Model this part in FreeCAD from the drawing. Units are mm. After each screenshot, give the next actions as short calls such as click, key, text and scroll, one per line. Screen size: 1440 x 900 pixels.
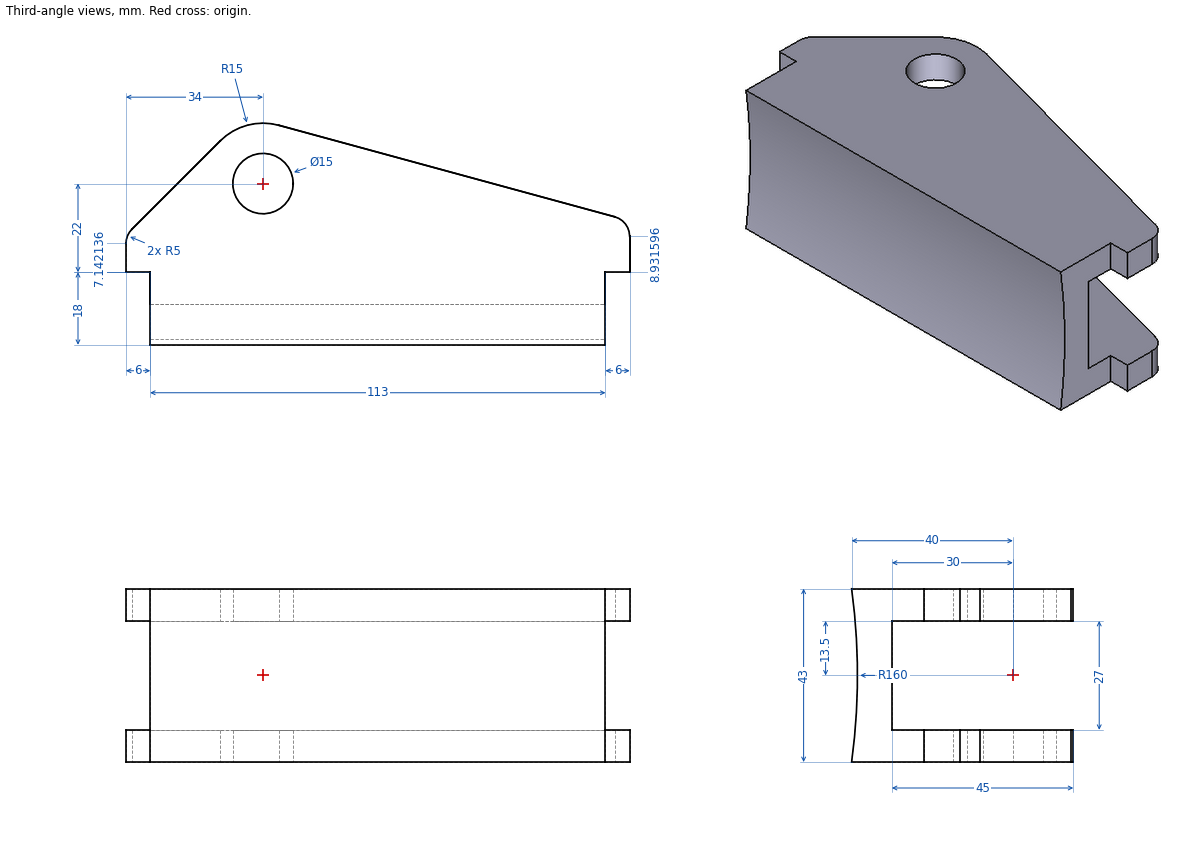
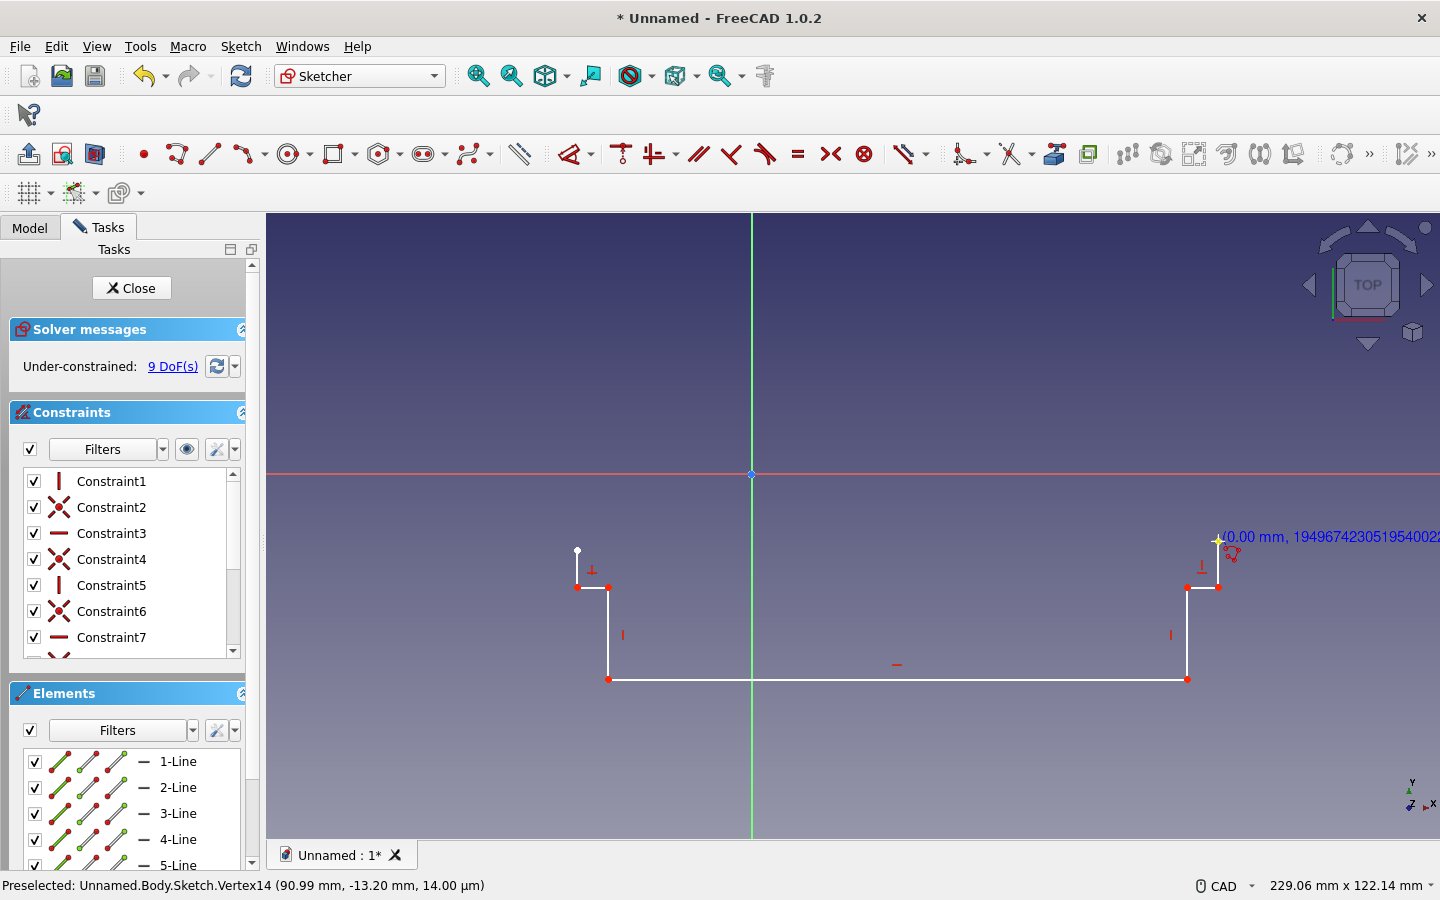
key(g)
key(l)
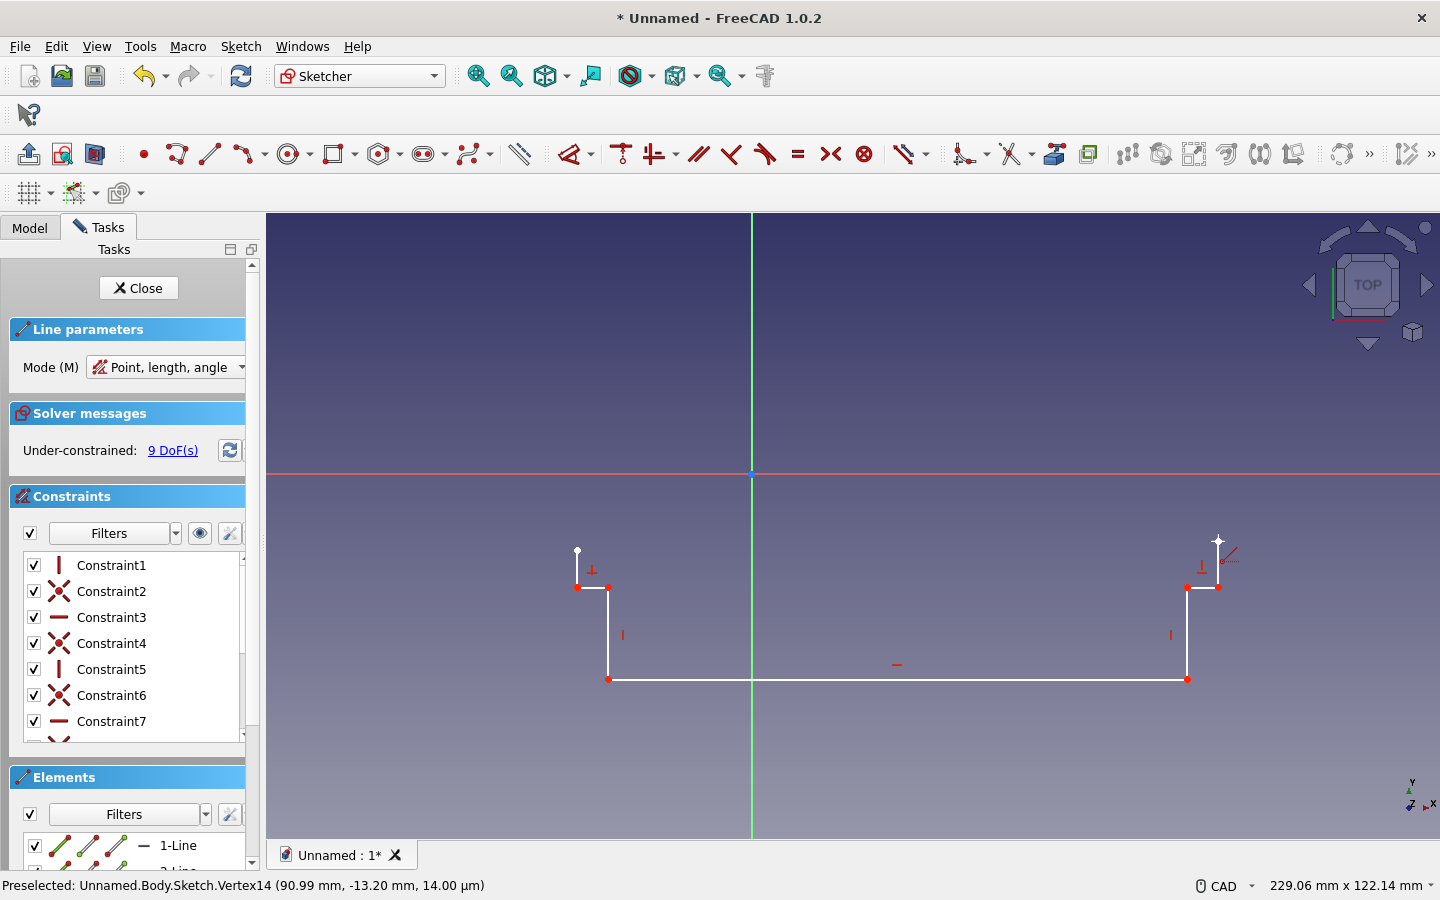
click(1199, 517)
click(772, 400)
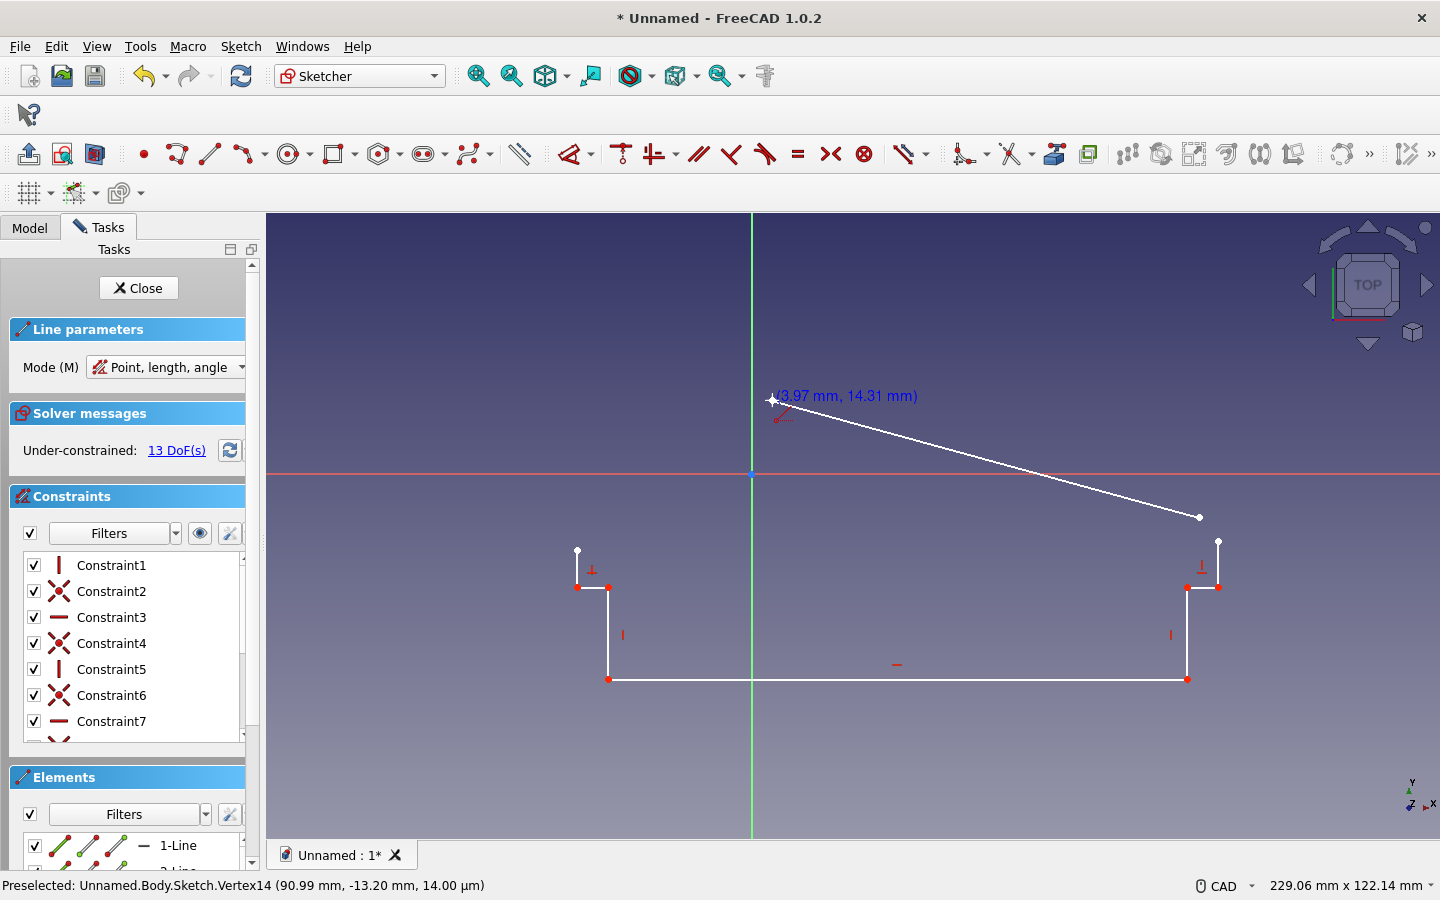
click(697, 420)
click(585, 532)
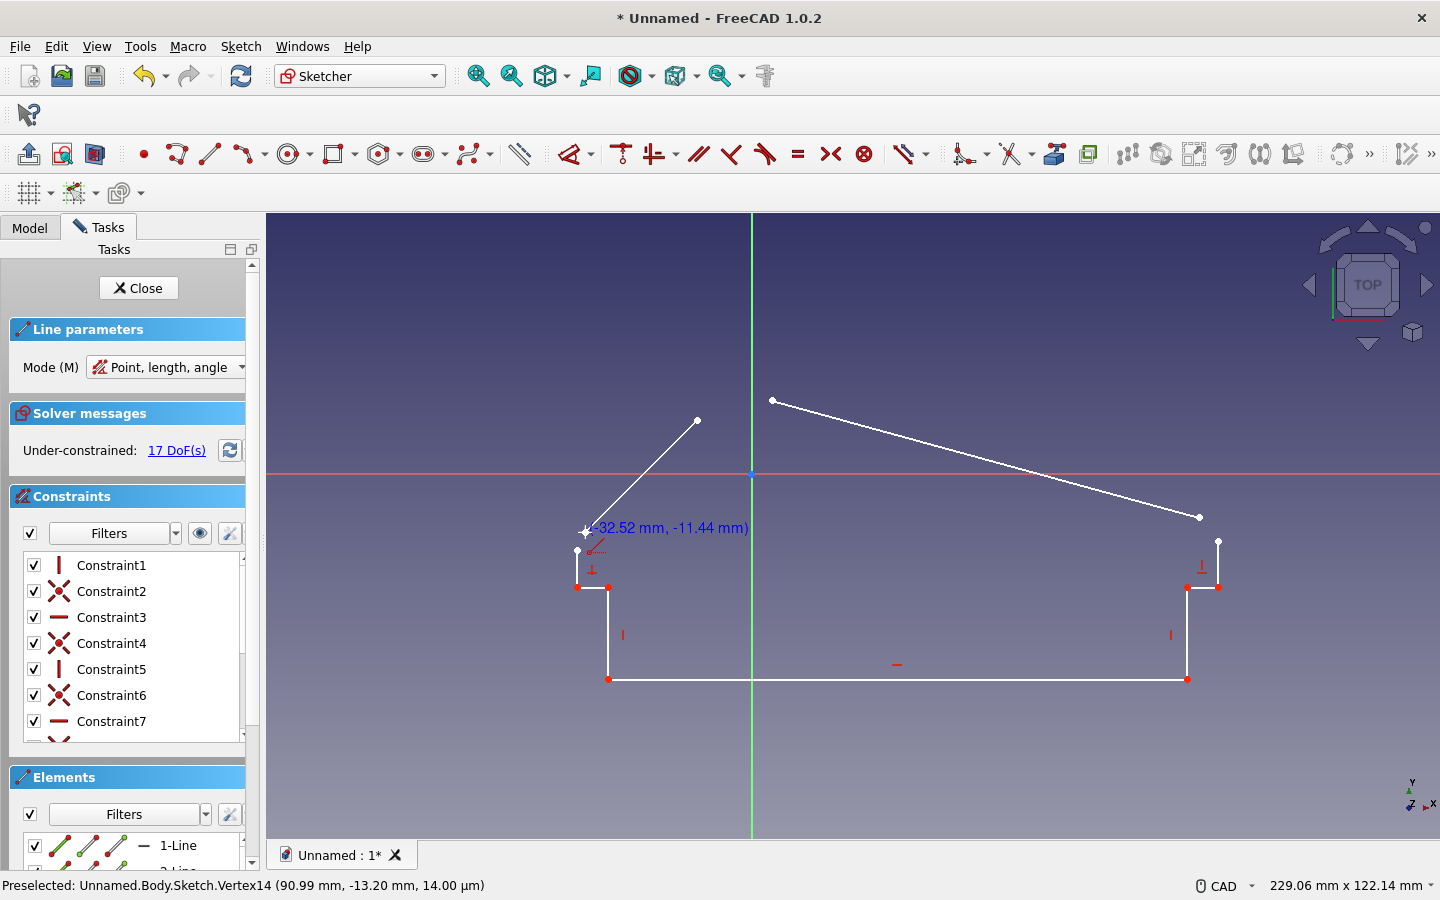
click(242, 154)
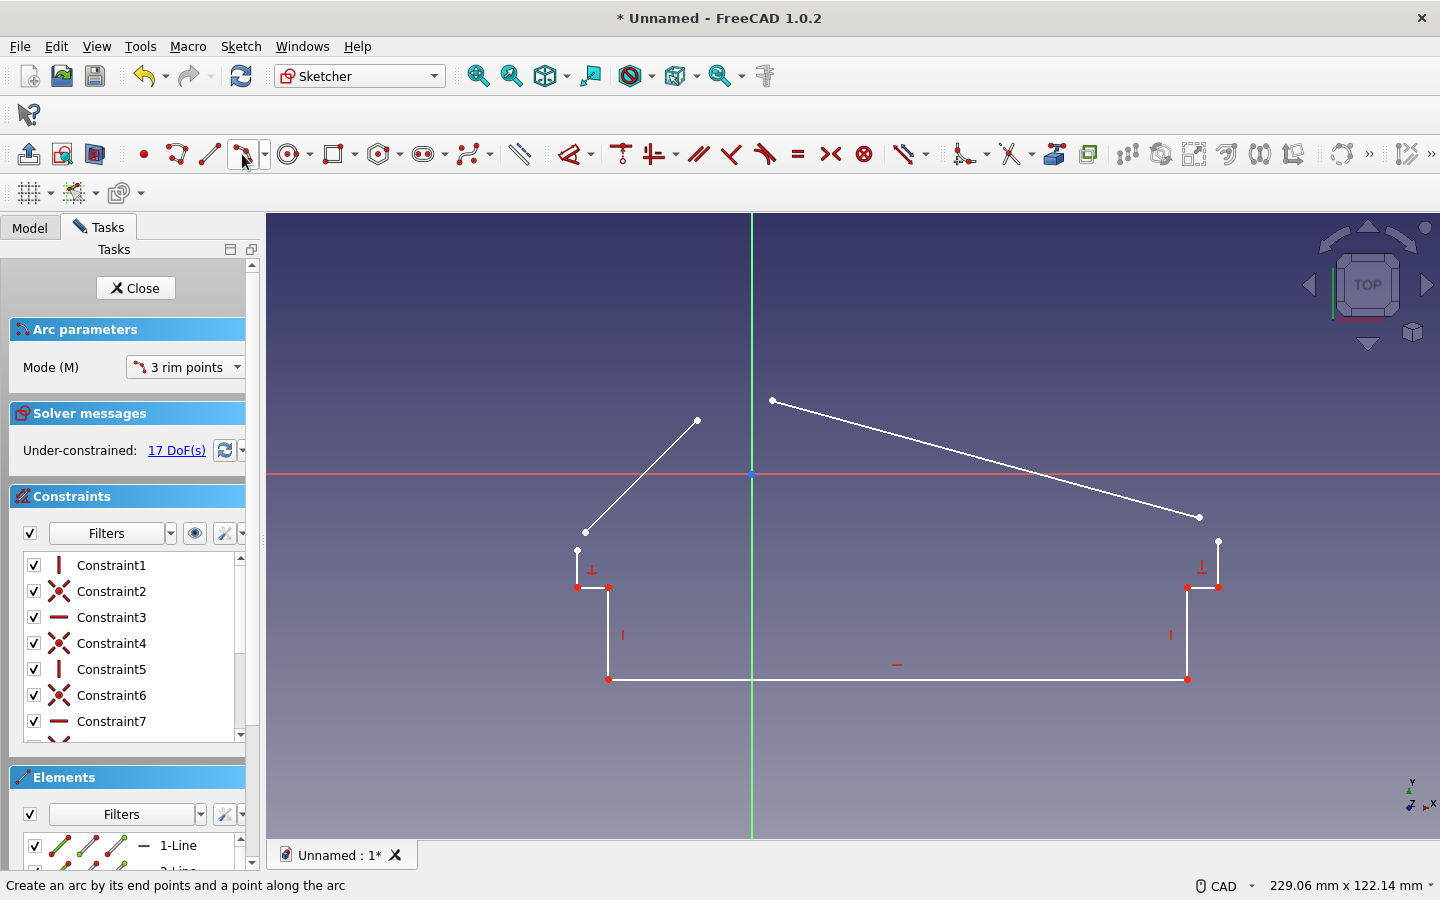
click(1218, 542)
click(1199, 518)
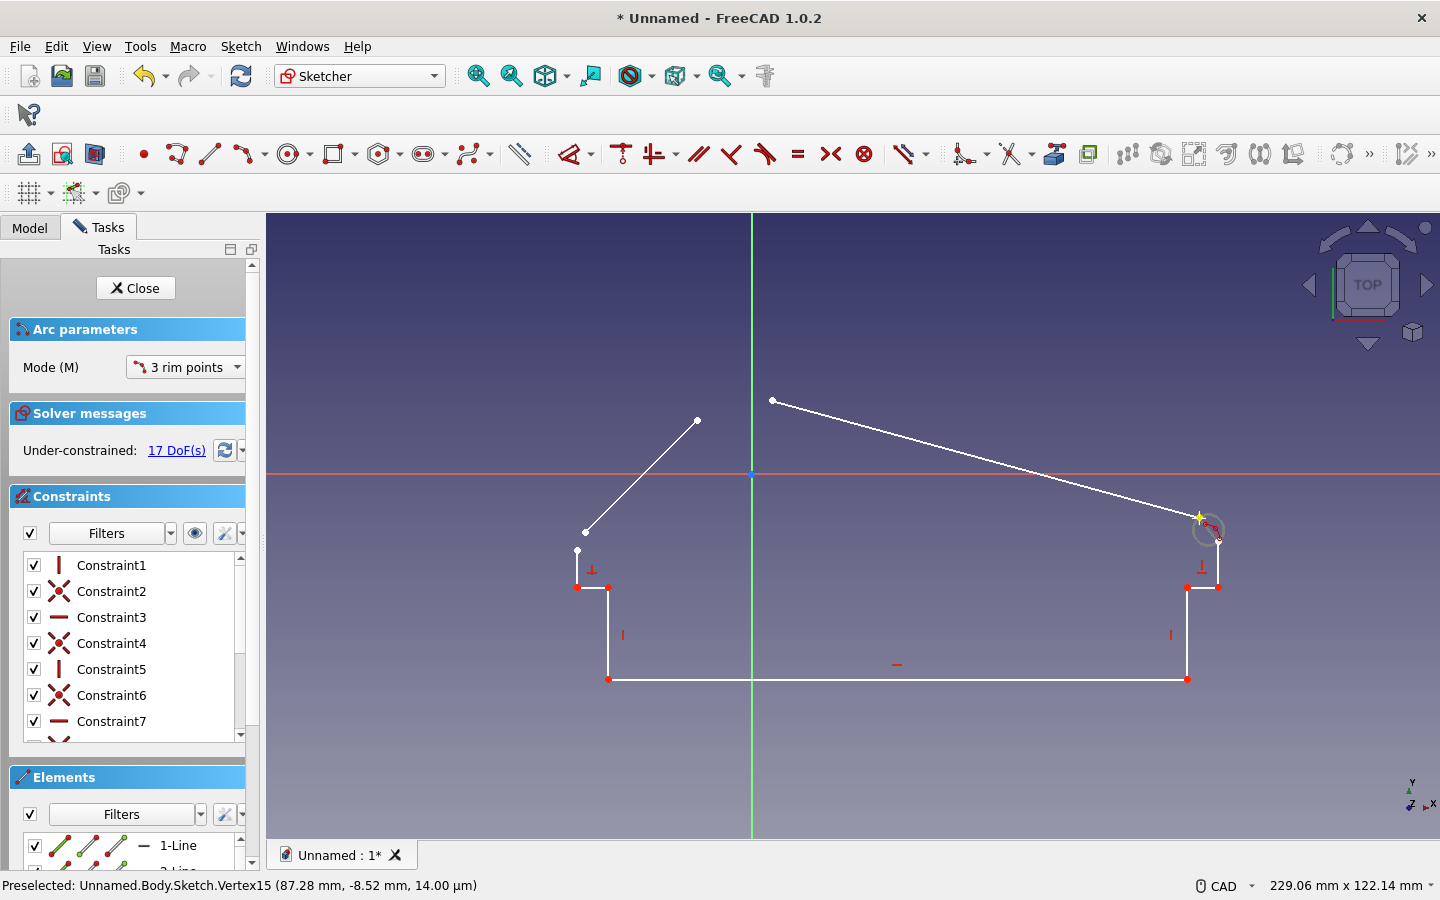
scroll(1213, 526, up, 6)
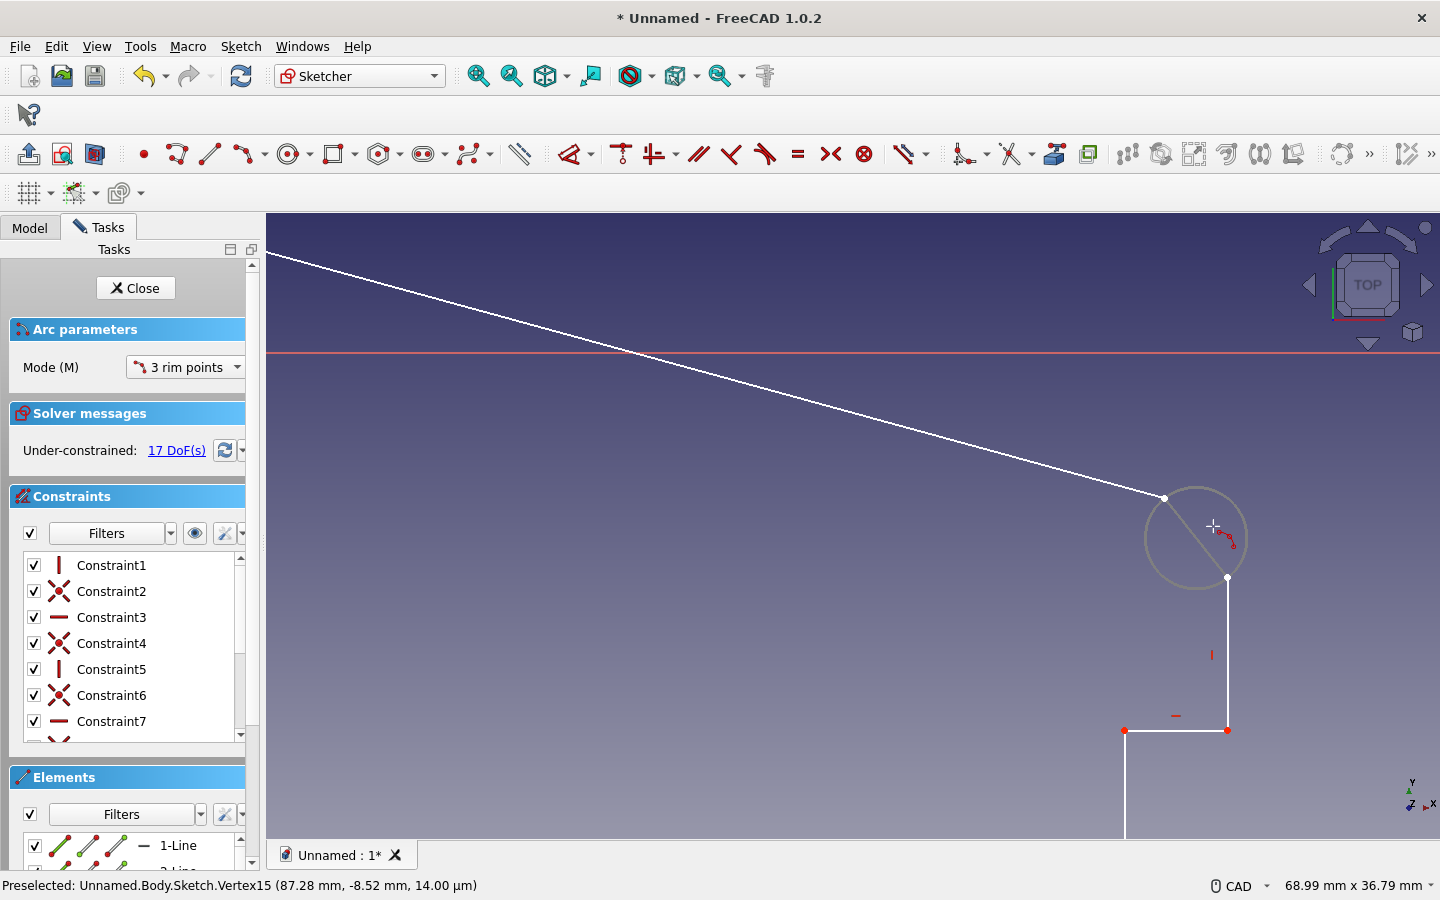
click(1210, 524)